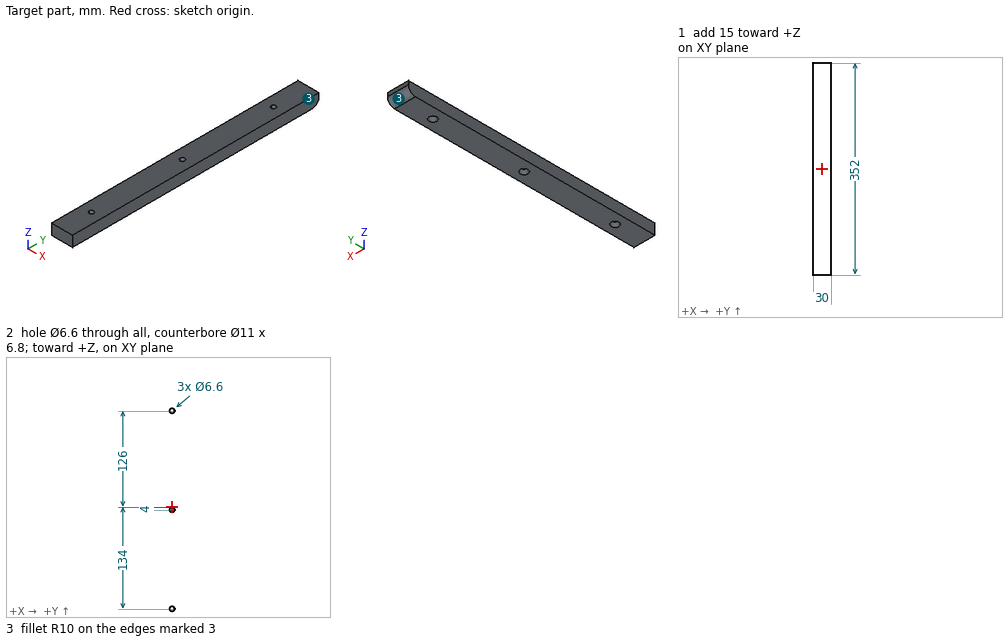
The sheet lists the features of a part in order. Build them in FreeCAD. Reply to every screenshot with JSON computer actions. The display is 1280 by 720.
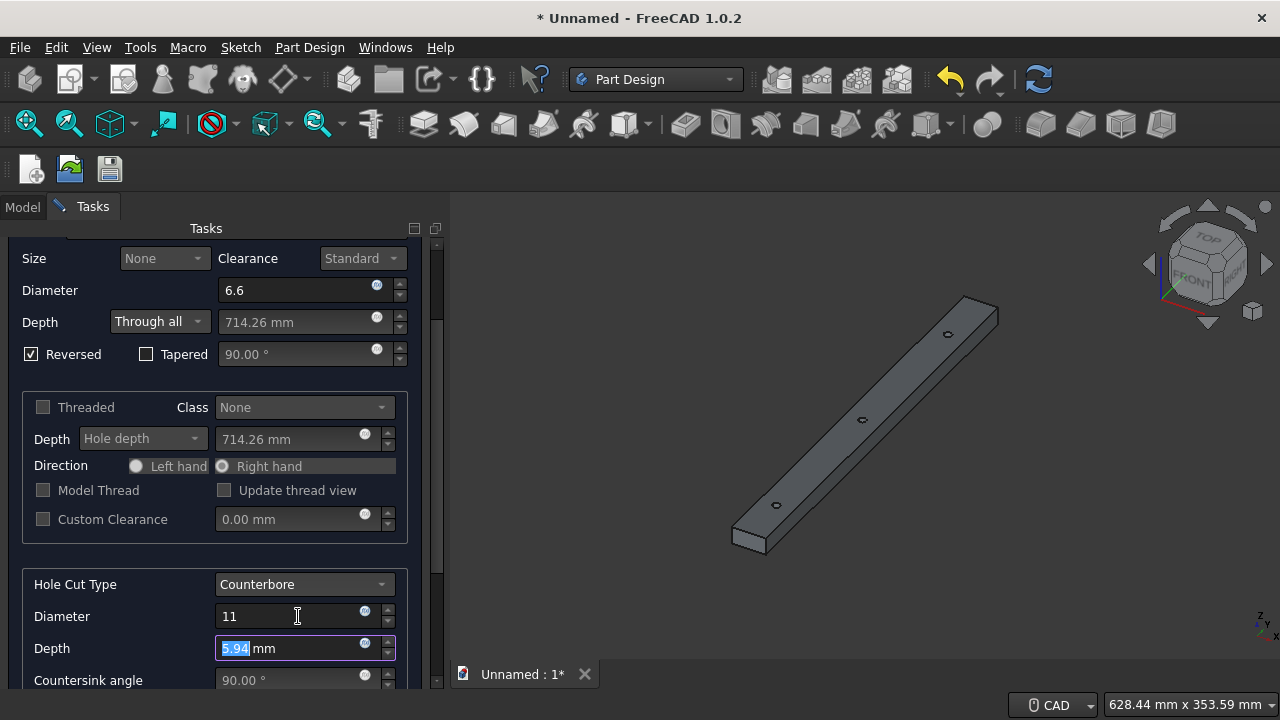
{"action": "type", "text": "6.8"}
{"action": "key", "text": "Tab"}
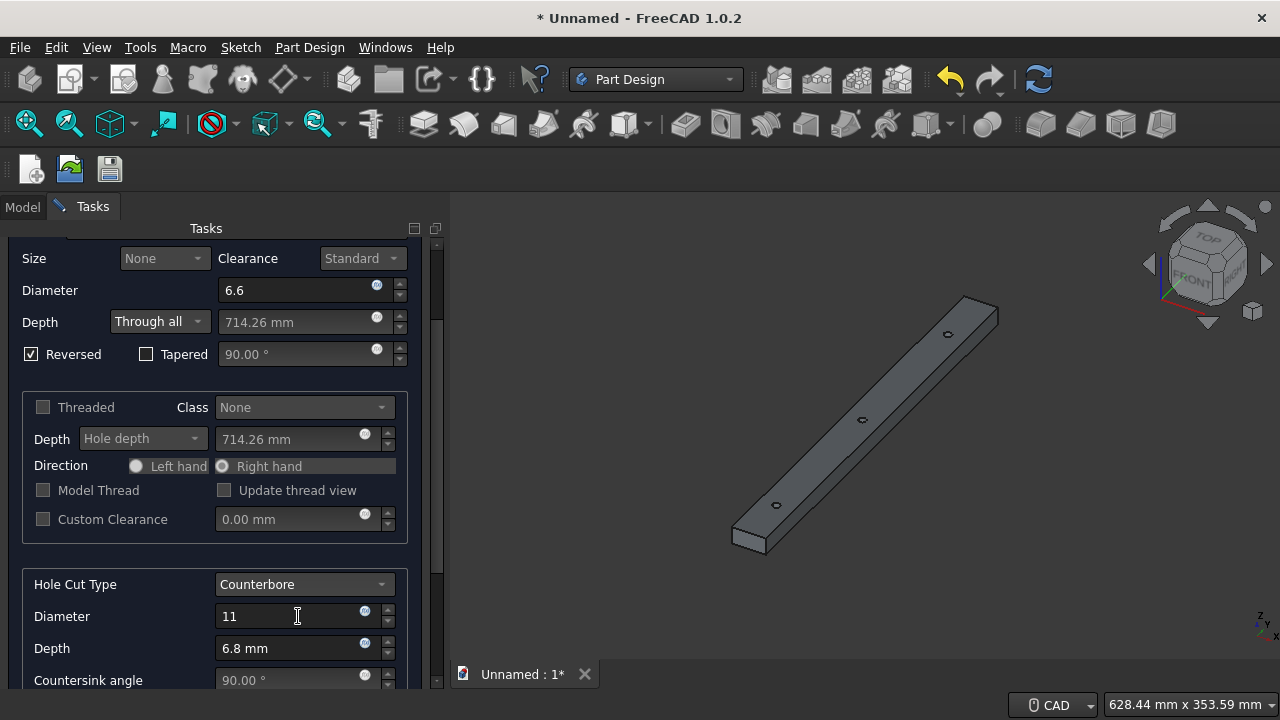
{"action": "scroll", "coordinate": [437, 463], "scroll_direction": "up", "scroll_amount": 3}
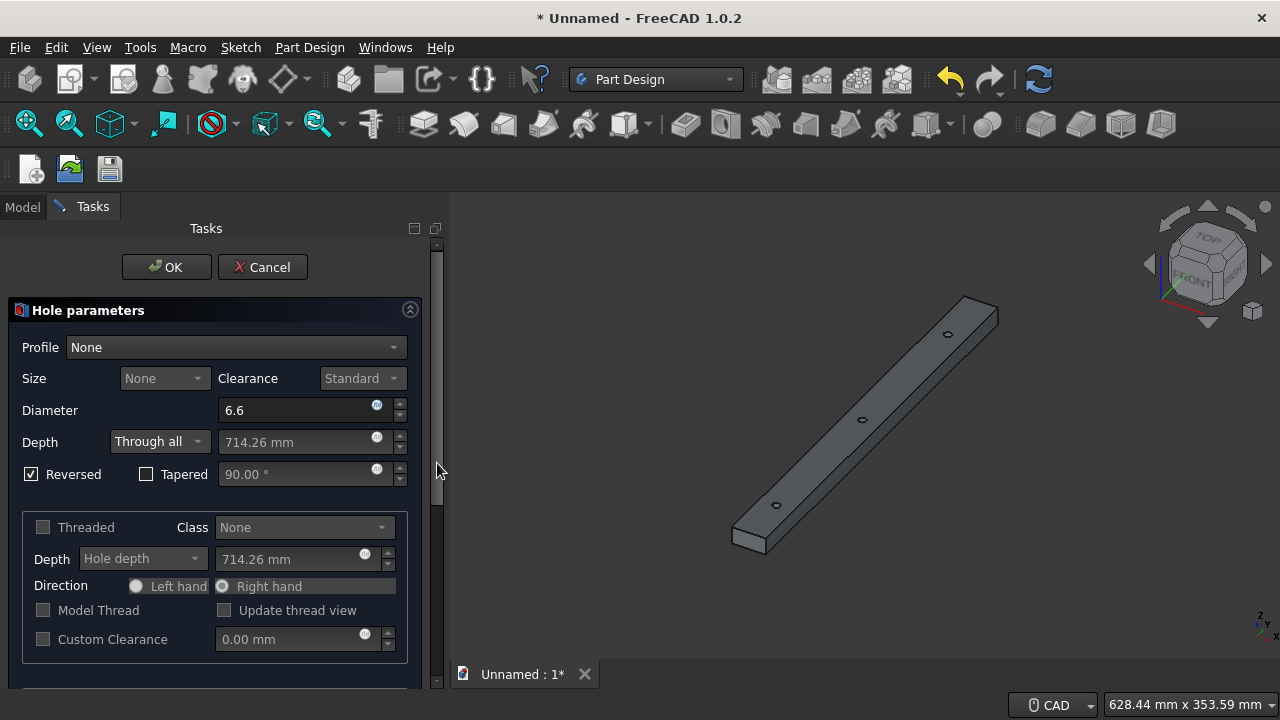
{"action": "left_click", "coordinate": [167, 267]}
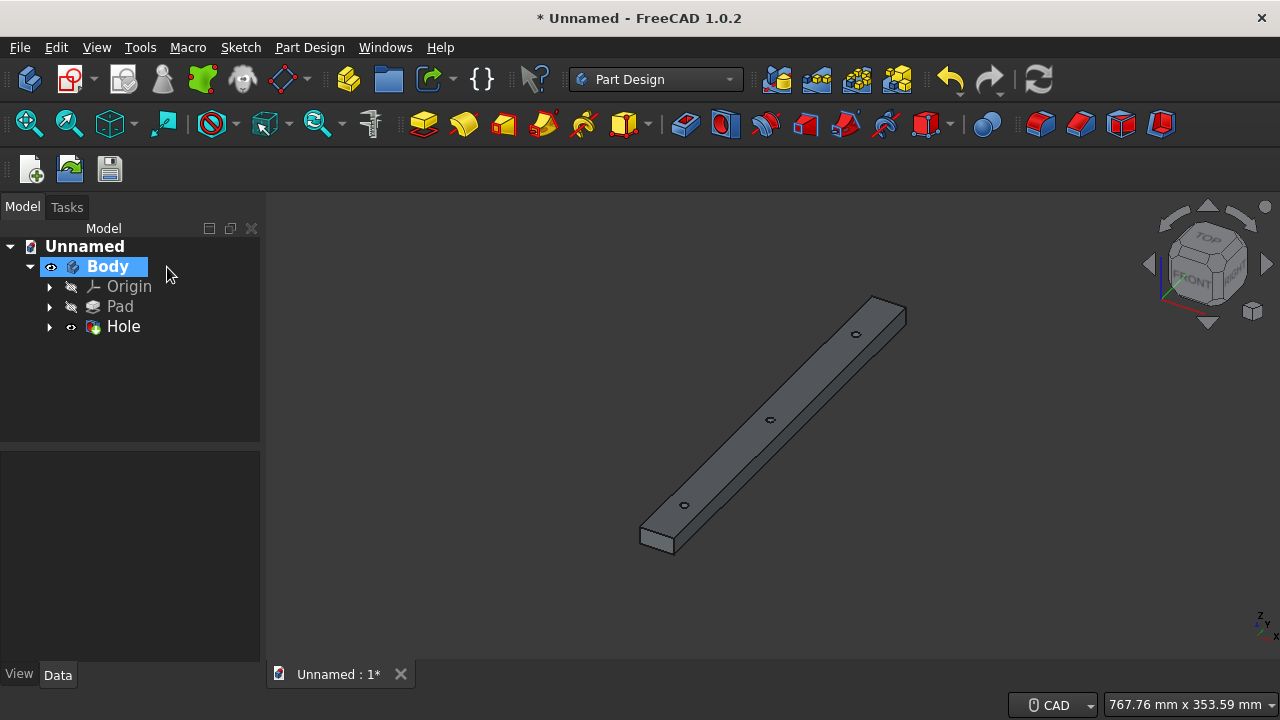
{"action": "key", "text": "0"}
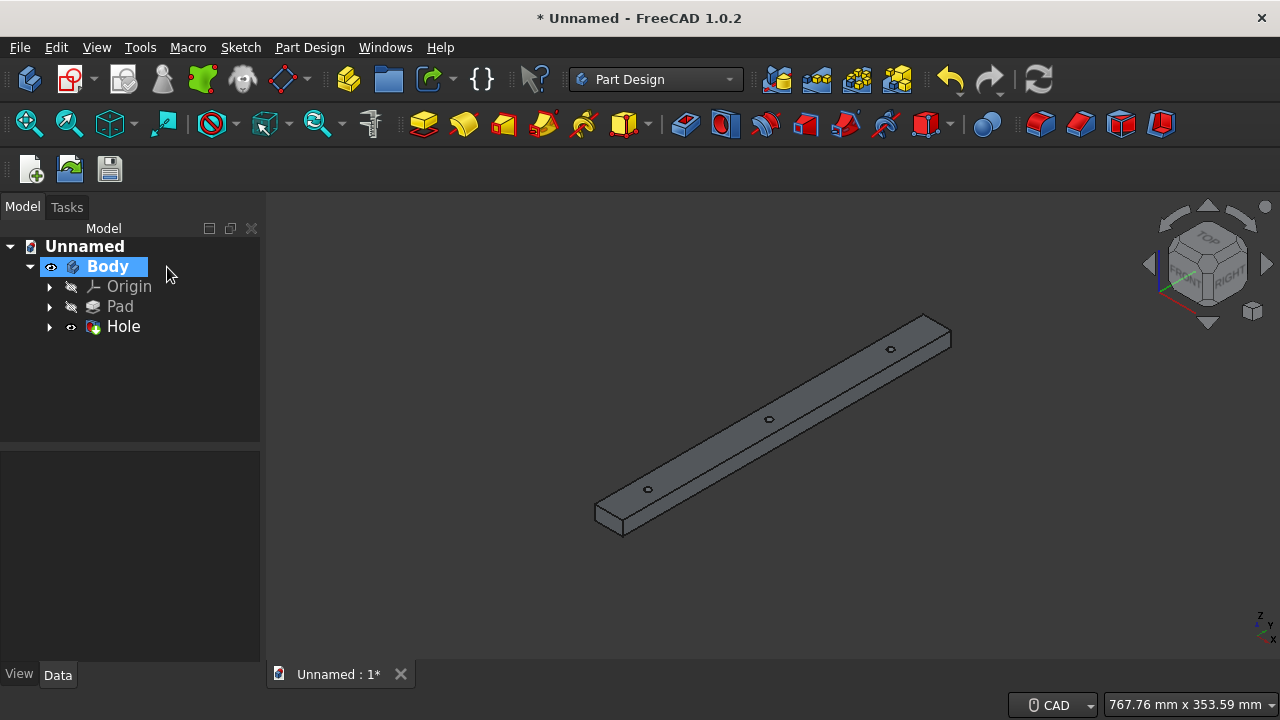
{"action": "key", "text": "2"}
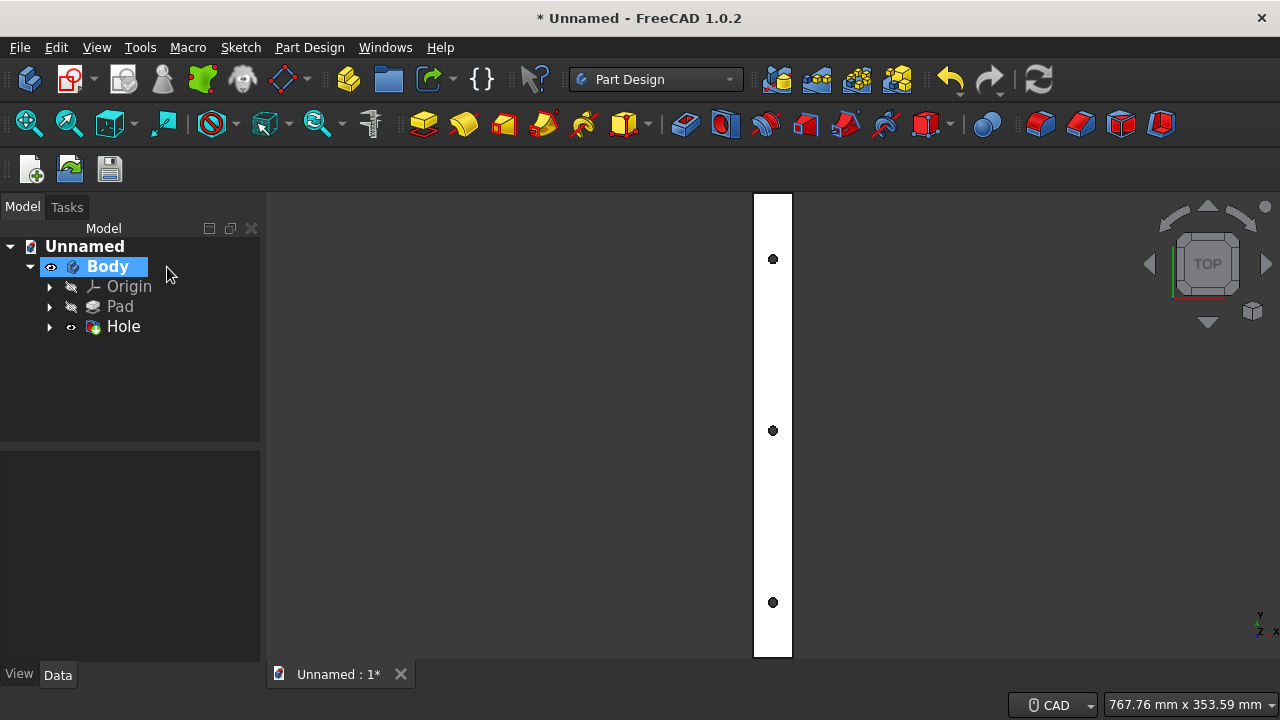
{"action": "key", "text": "1"}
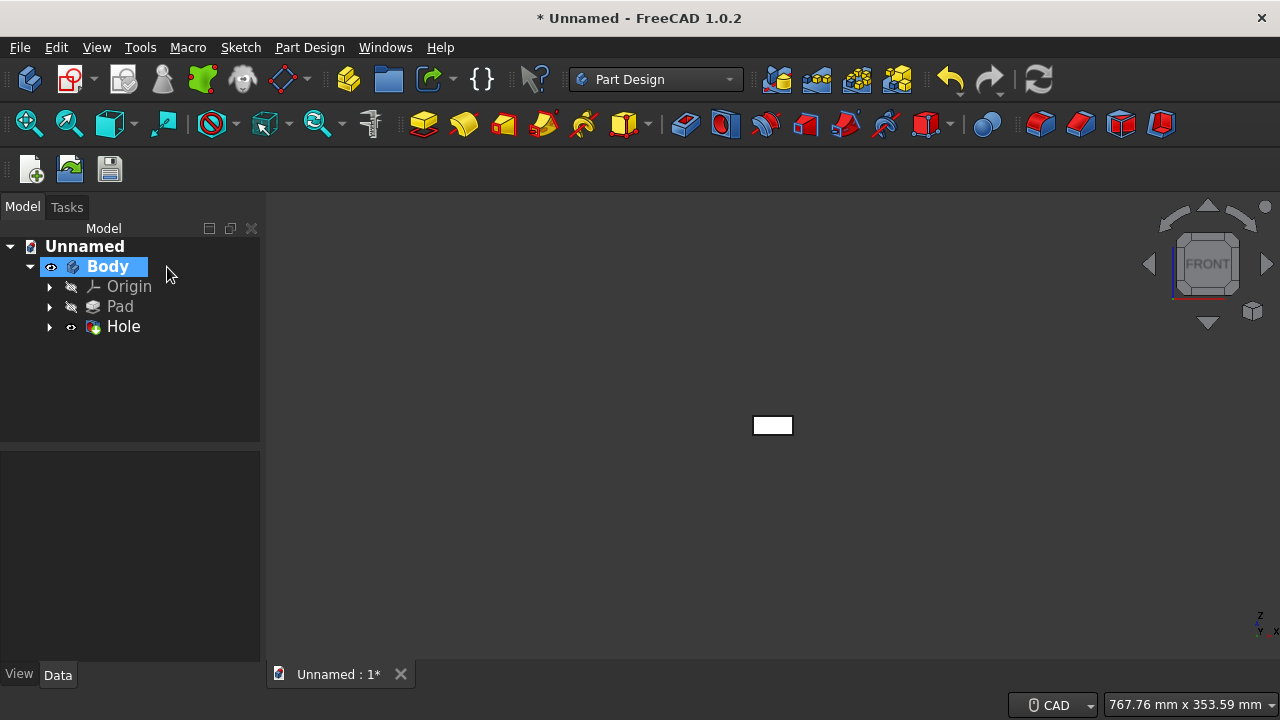
{"action": "left_click", "coordinate": [30, 124]}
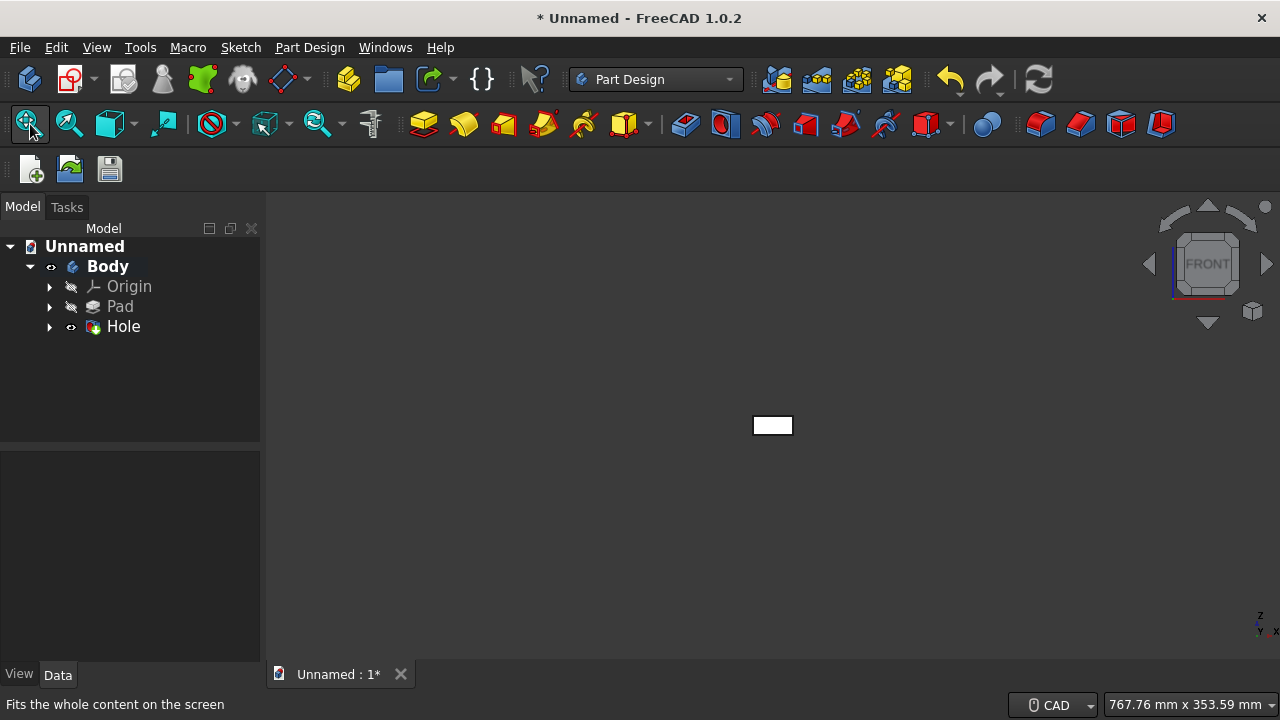
{"action": "key", "text": "3"}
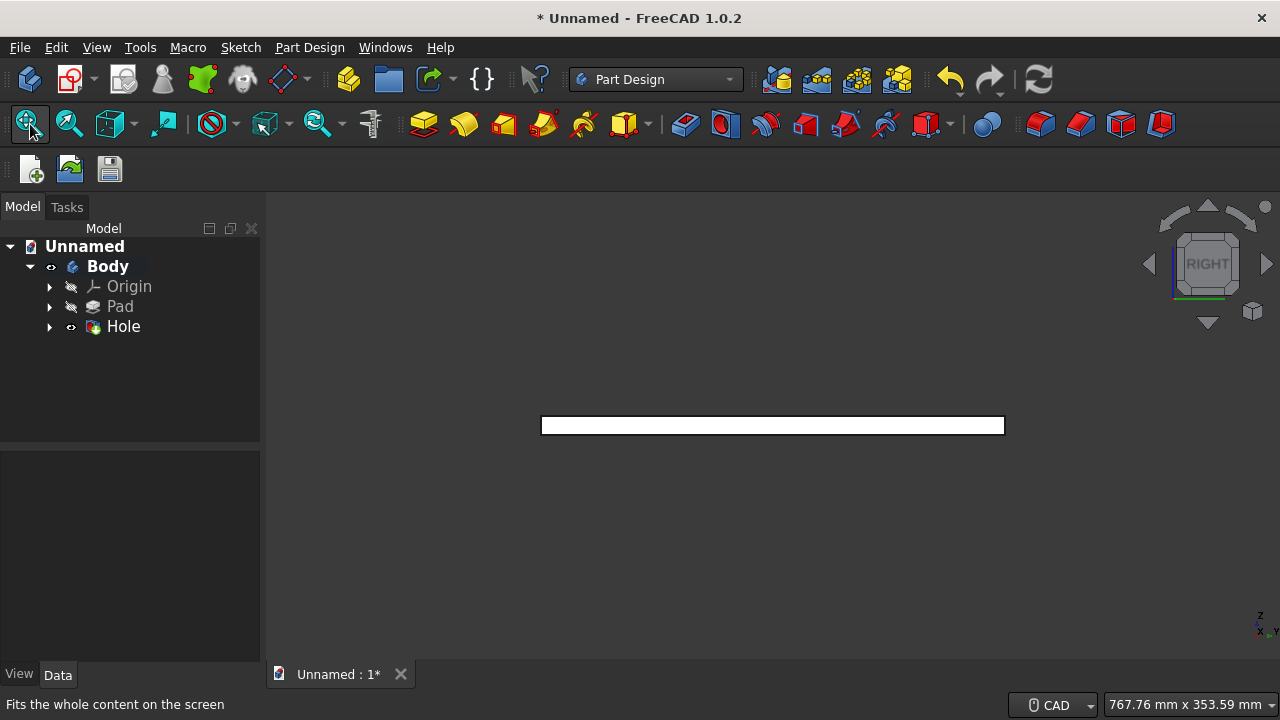
{"action": "key", "text": "5"}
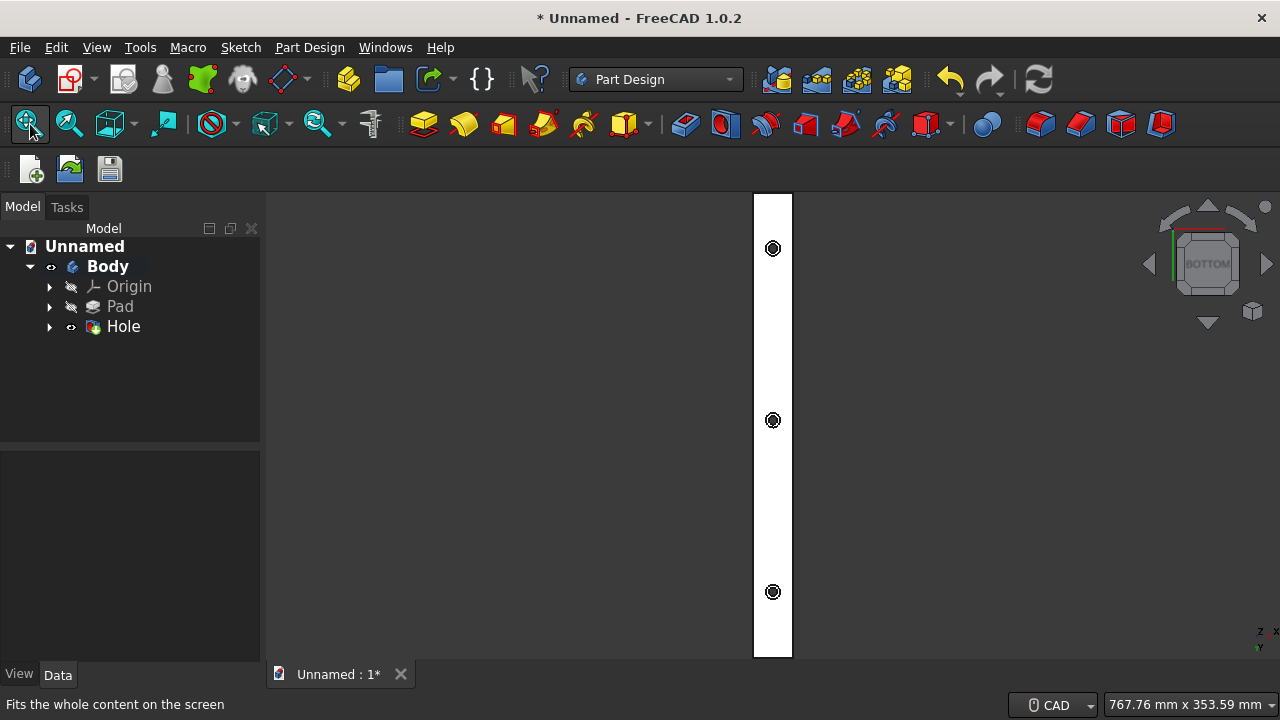
{"action": "key", "text": "4"}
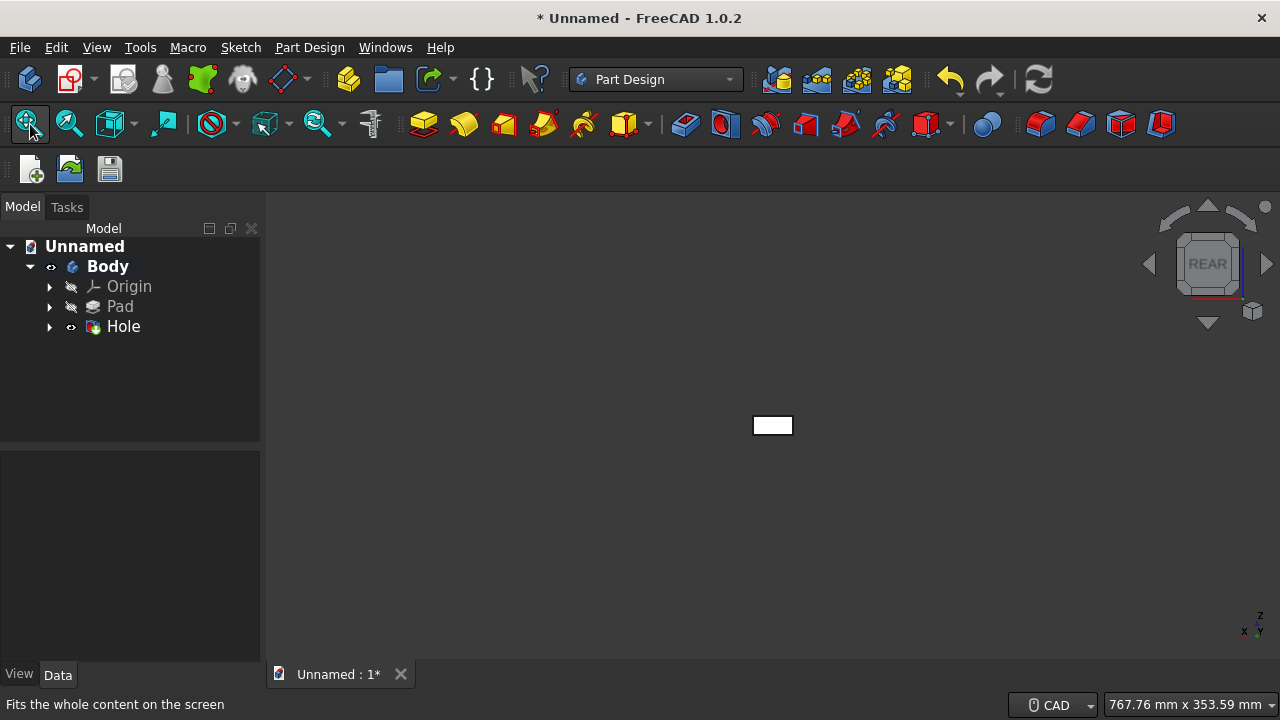
{"action": "left_click", "coordinate": [30, 124]}